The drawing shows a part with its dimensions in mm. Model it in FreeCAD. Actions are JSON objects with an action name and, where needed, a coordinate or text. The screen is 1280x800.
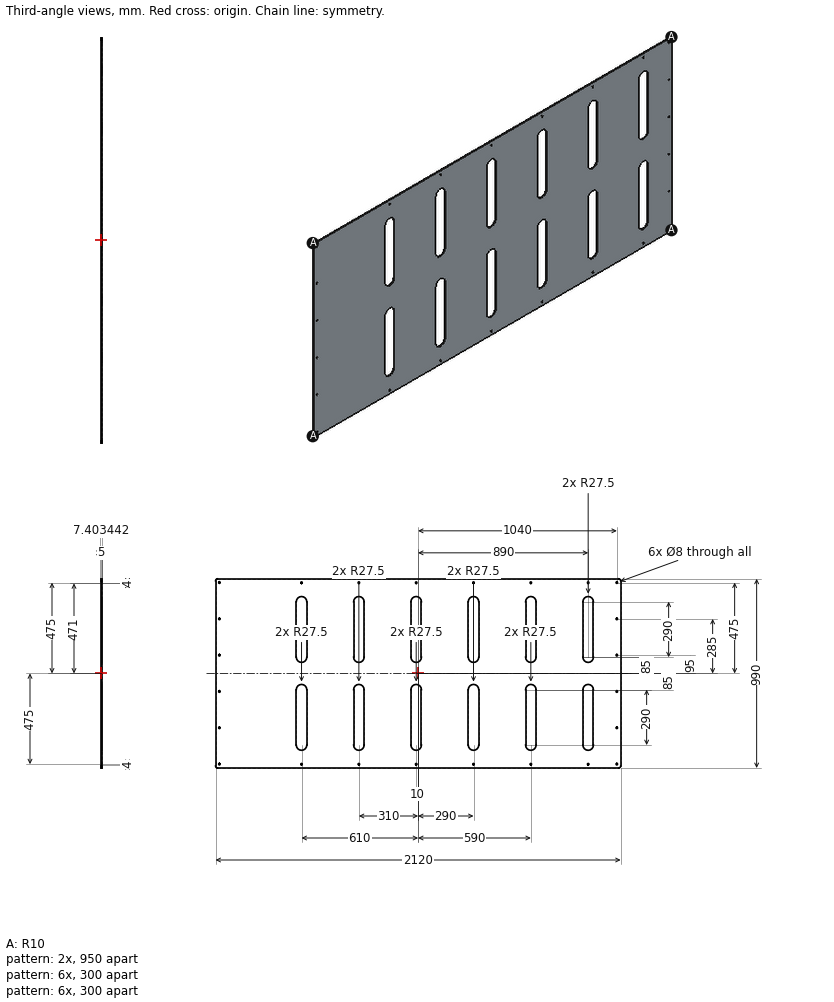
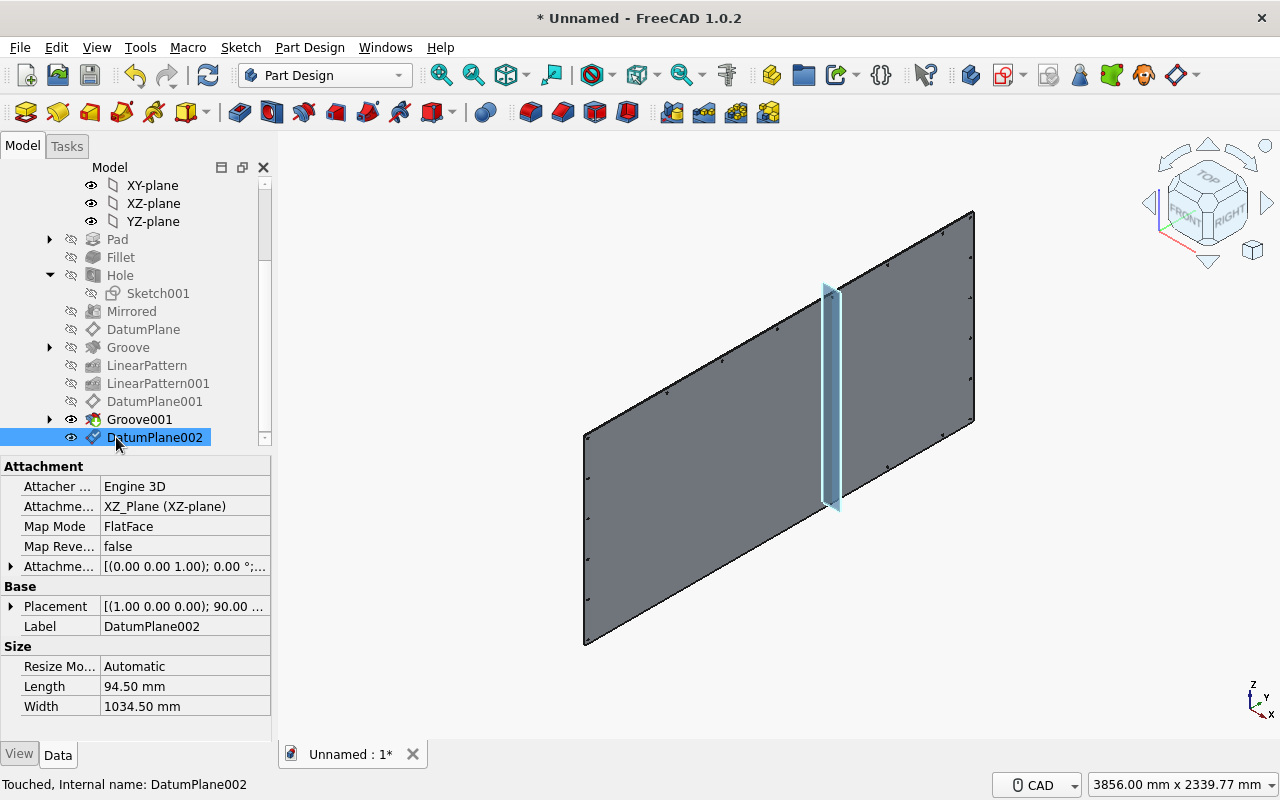
{"action": "left_click", "coordinate": [1004, 76]}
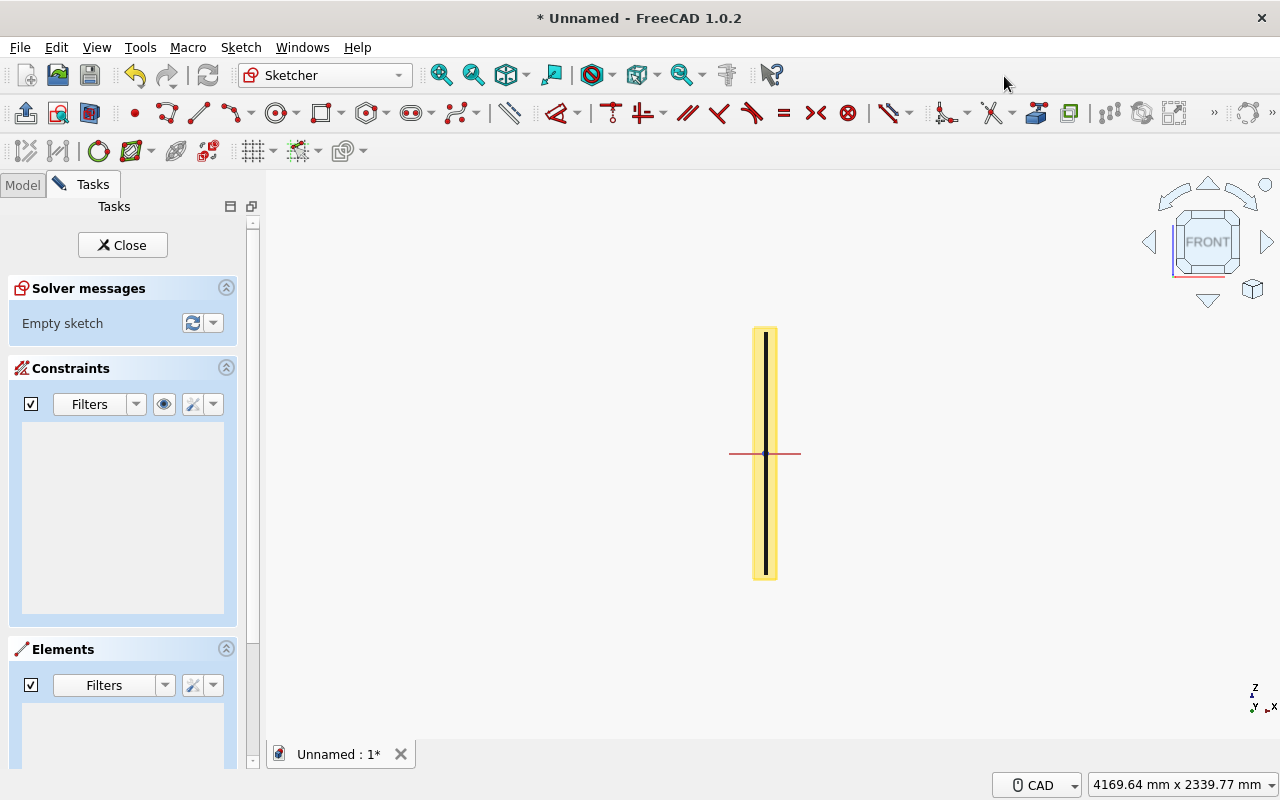
{"action": "key", "text": "q s"}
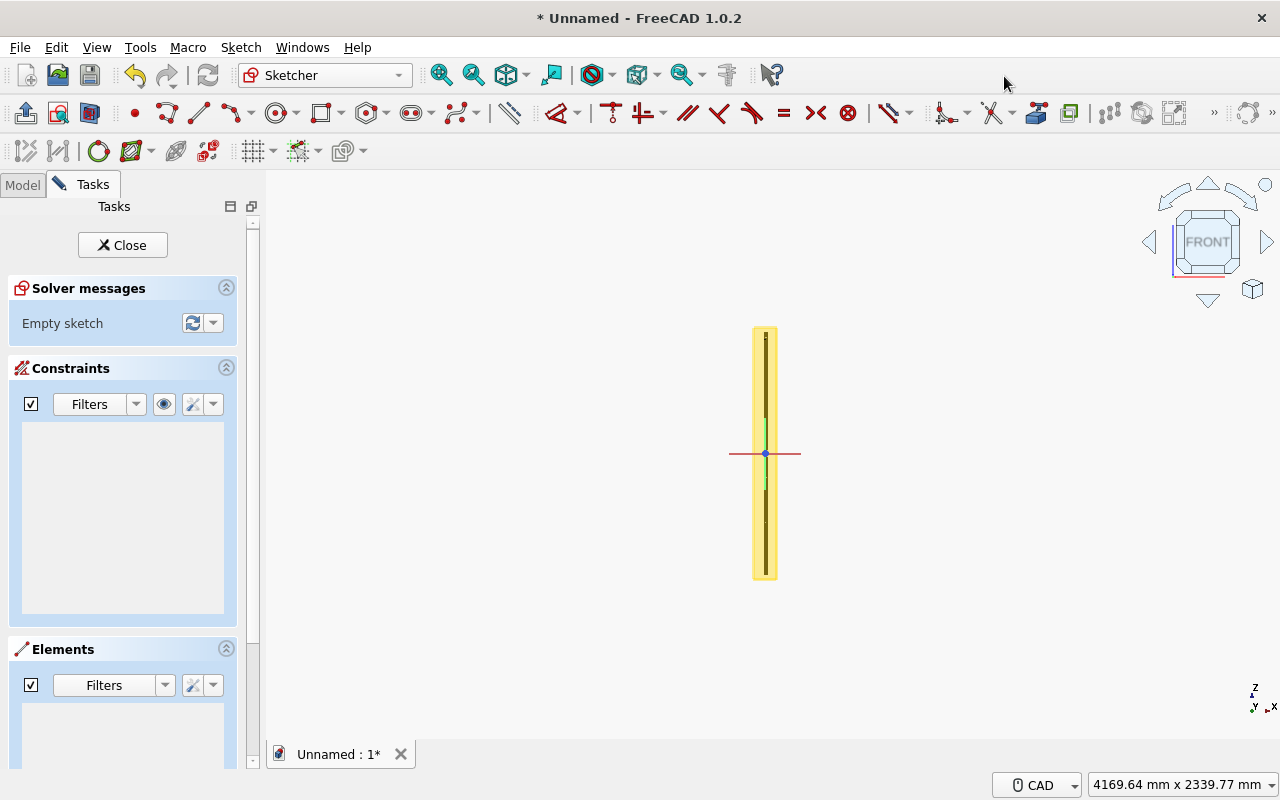
{"action": "scroll", "coordinate": [769, 576], "scroll_direction": "up", "scroll_amount": 15}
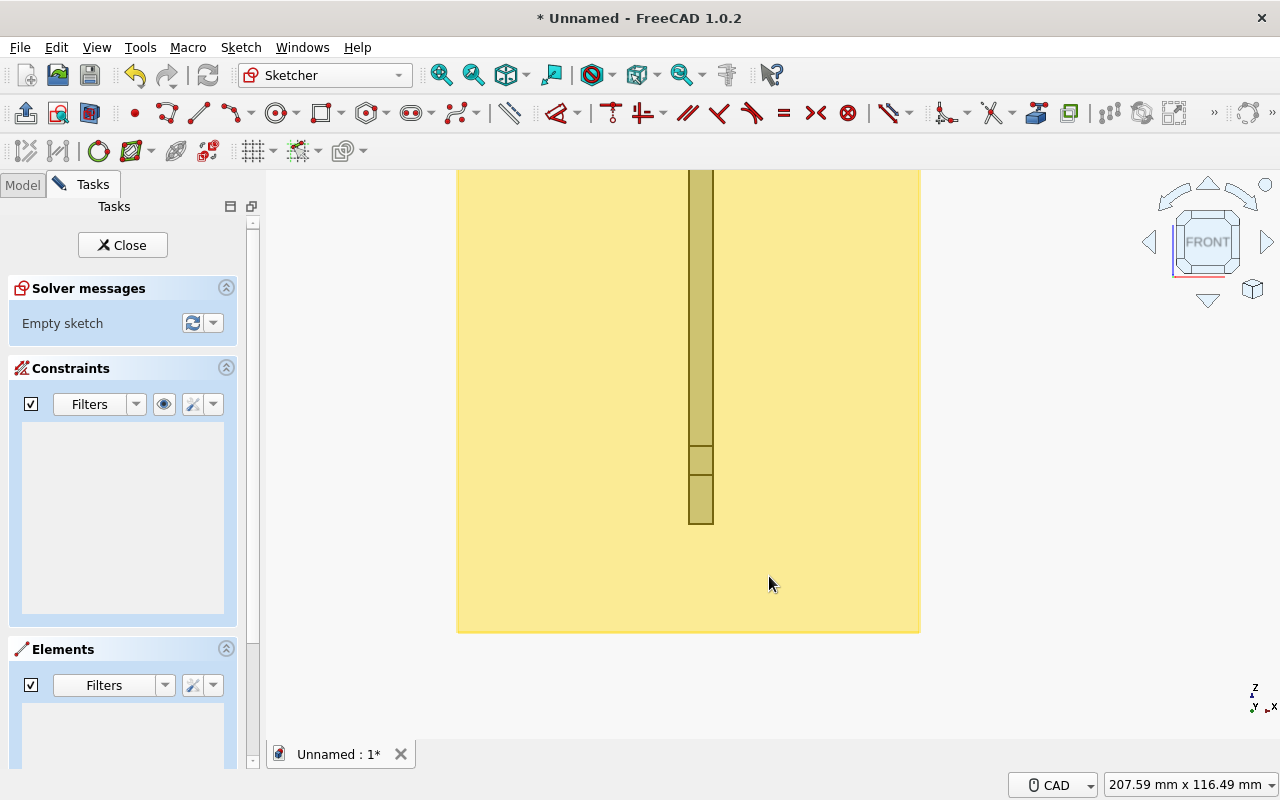
{"action": "scroll", "coordinate": [686, 434], "scroll_direction": "up", "scroll_amount": 12}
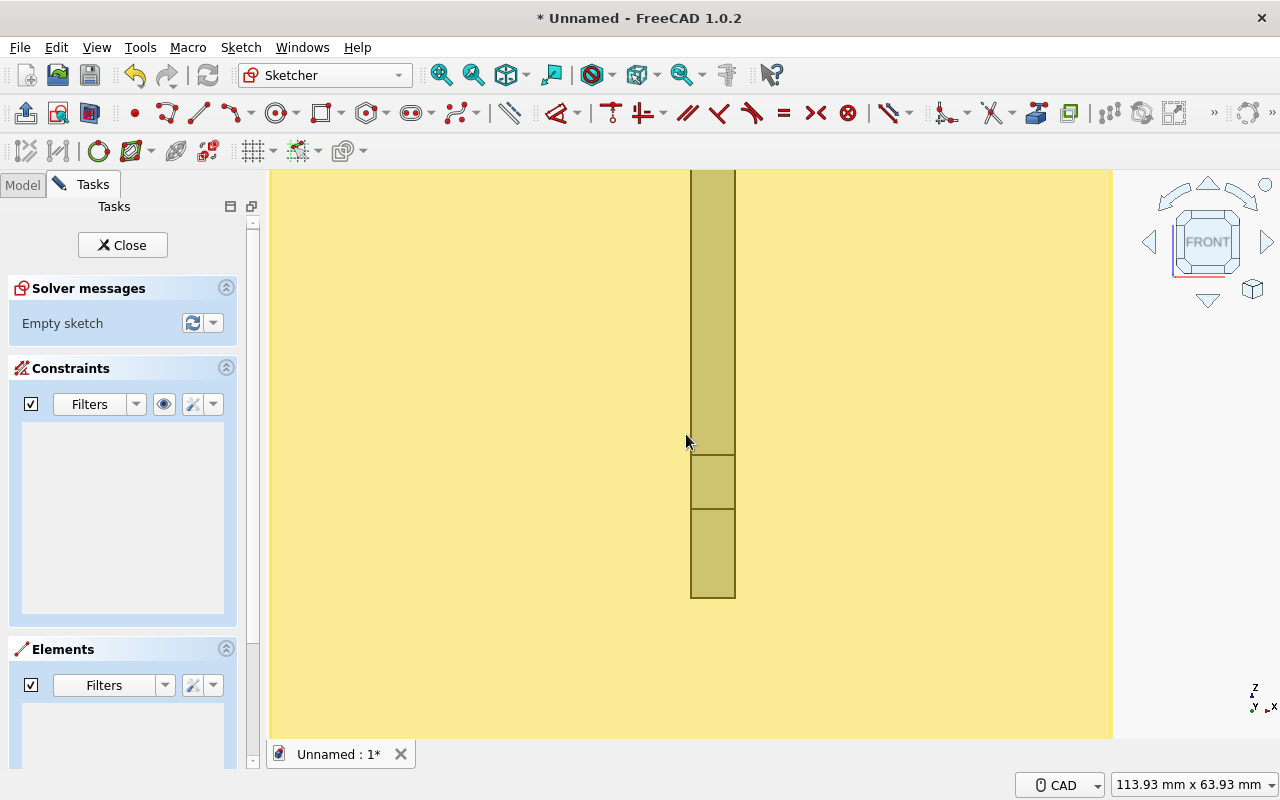
{"action": "left_click", "coordinate": [168, 114]}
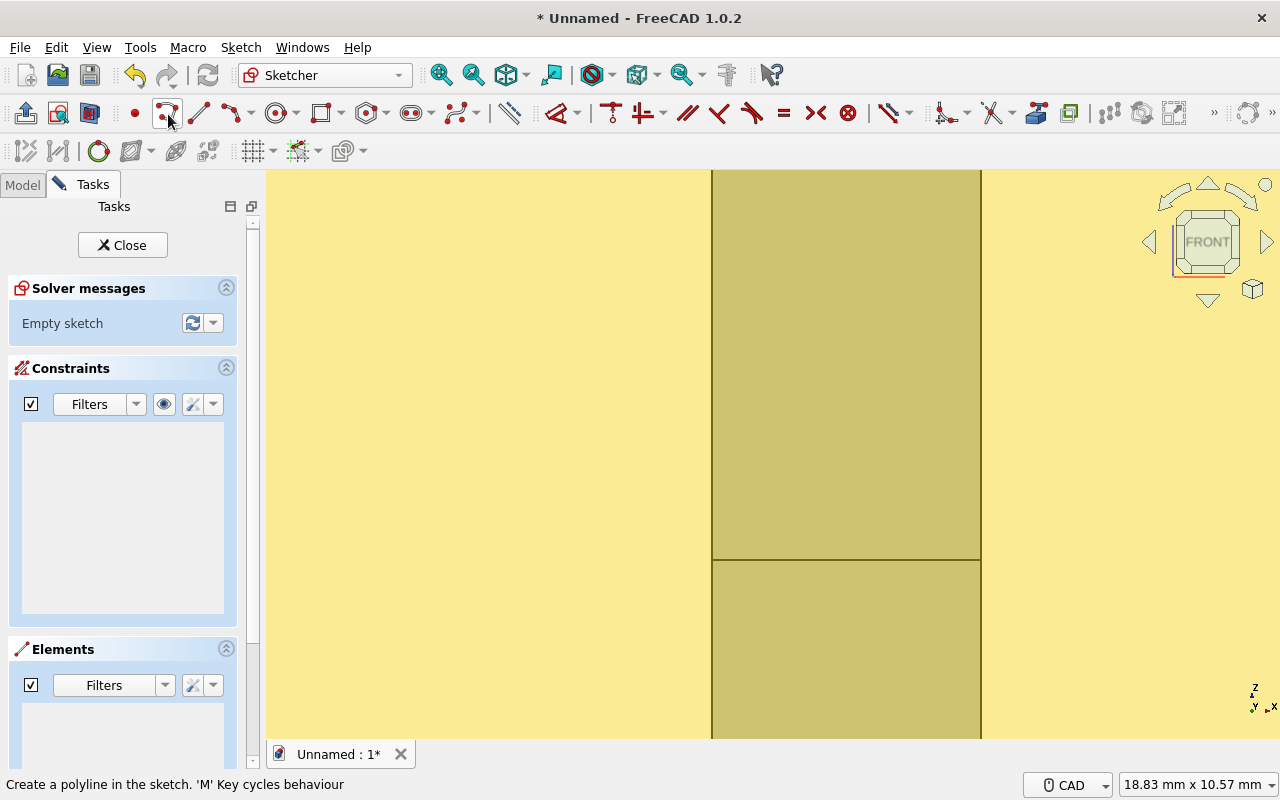
{"action": "left_click", "coordinate": [582, 345]}
{"action": "left_click", "coordinate": [981, 345]}
{"action": "left_click", "coordinate": [981, 560]}
{"action": "left_click", "coordinate": [712, 560]}
{"action": "left_click", "coordinate": [582, 346]}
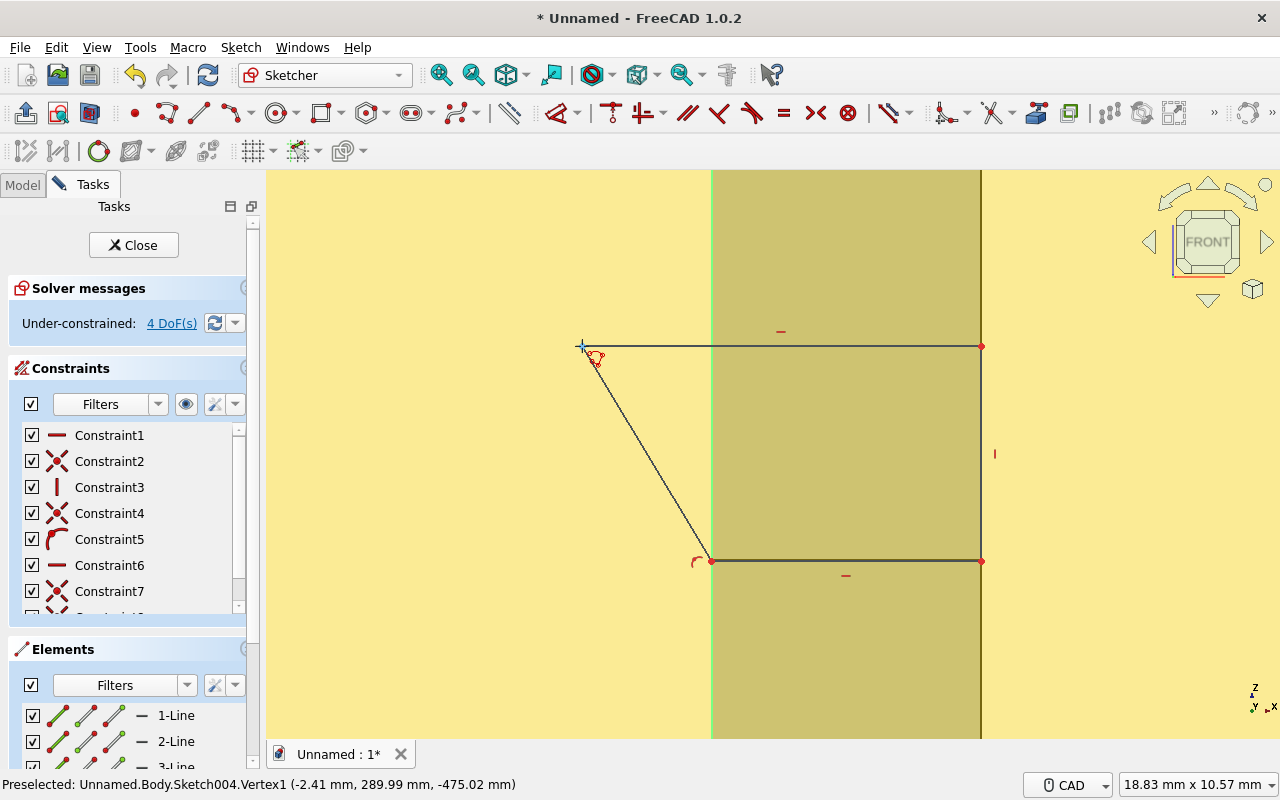
{"action": "key", "text": "g l"}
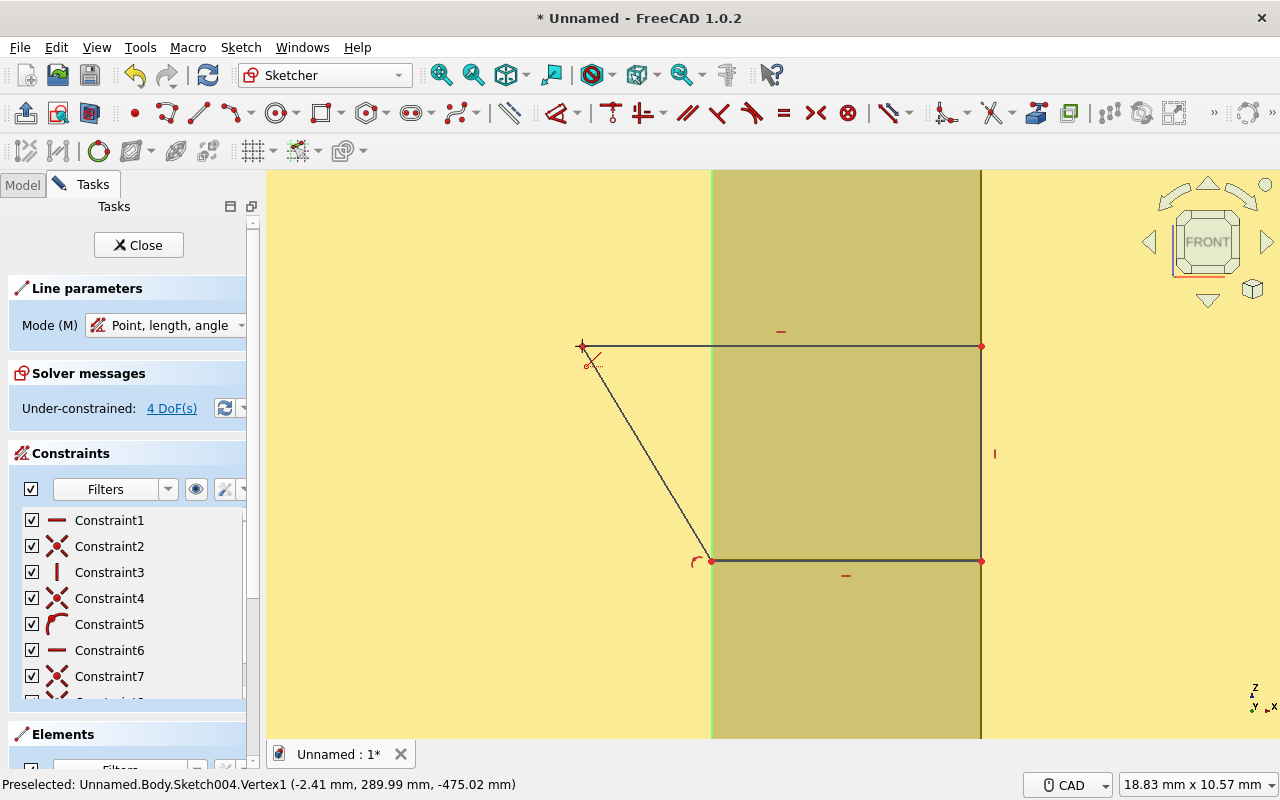
{"action": "left_click", "coordinate": [542, 345]}
{"action": "left_click", "coordinate": [423, 345]}
{"action": "key", "text": "Escape"}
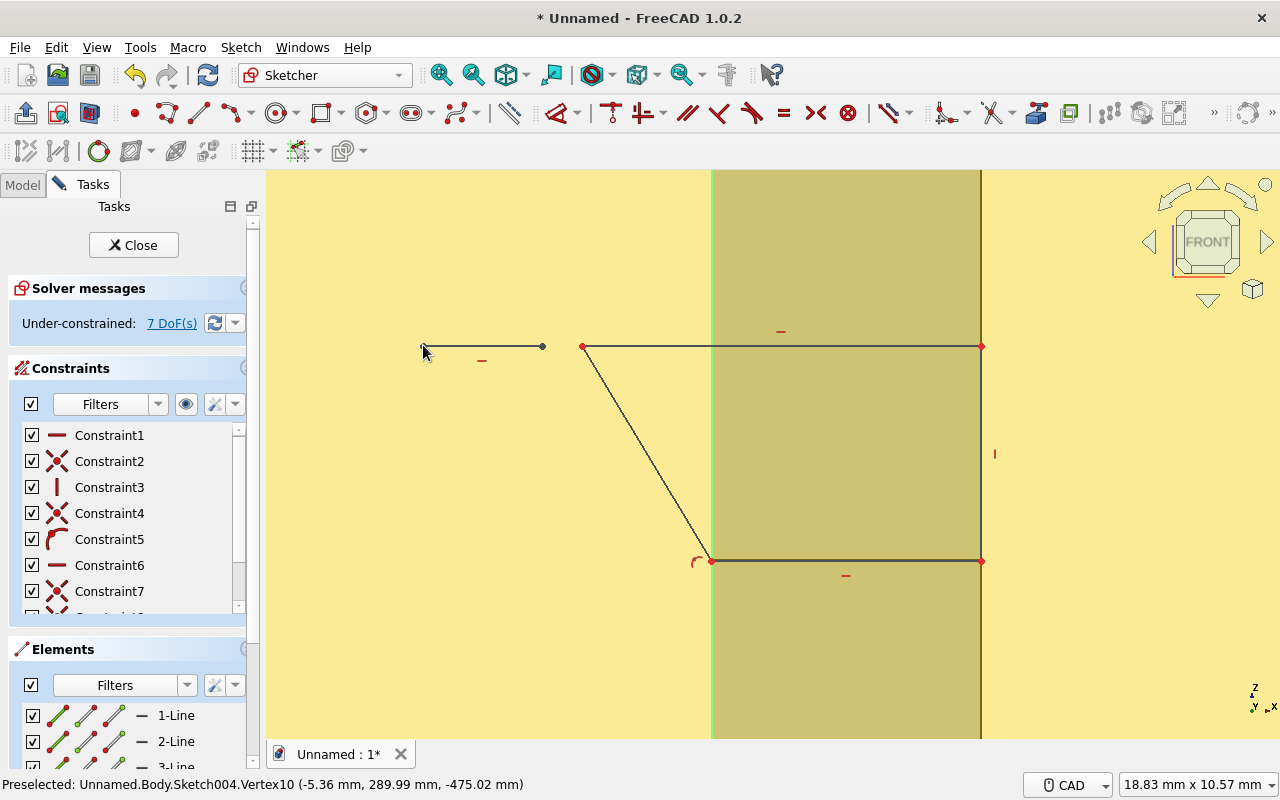
{"action": "left_click", "coordinate": [506, 346]}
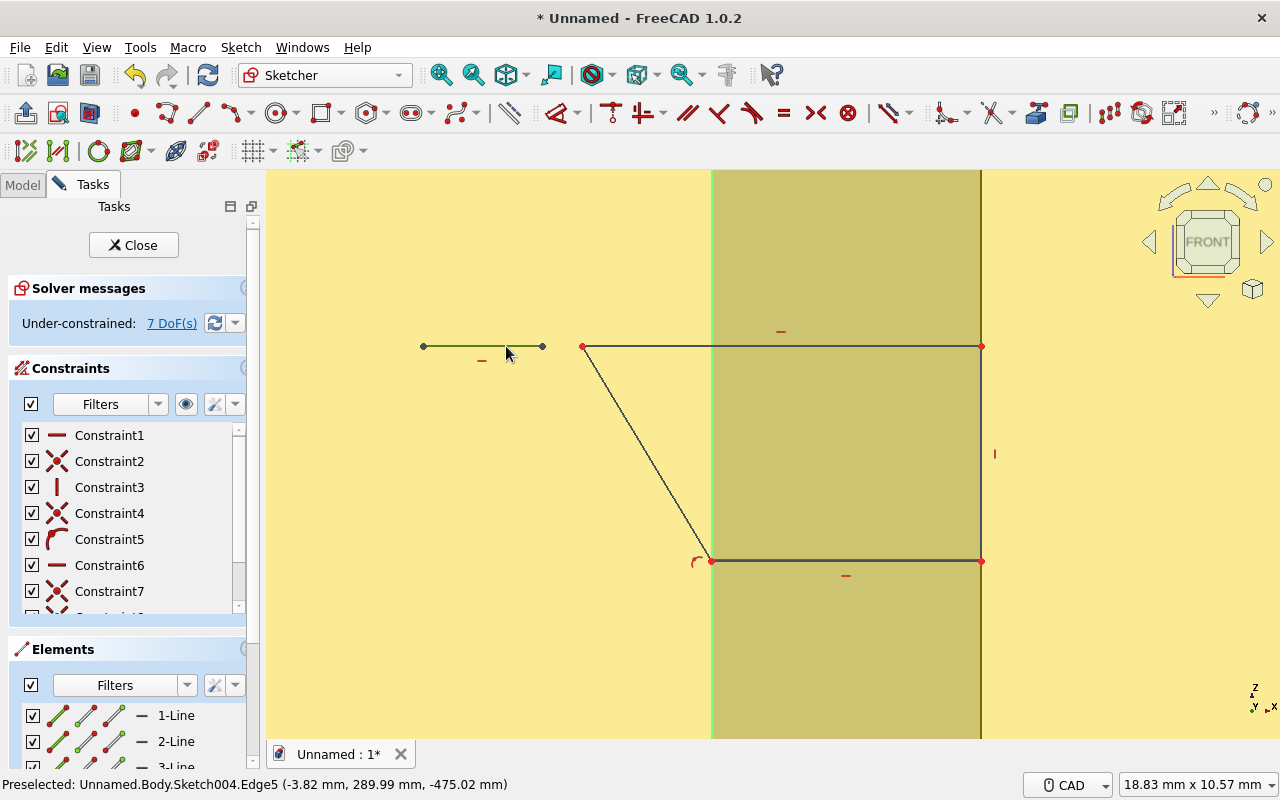
{"action": "left_click", "coordinate": [510, 114]}